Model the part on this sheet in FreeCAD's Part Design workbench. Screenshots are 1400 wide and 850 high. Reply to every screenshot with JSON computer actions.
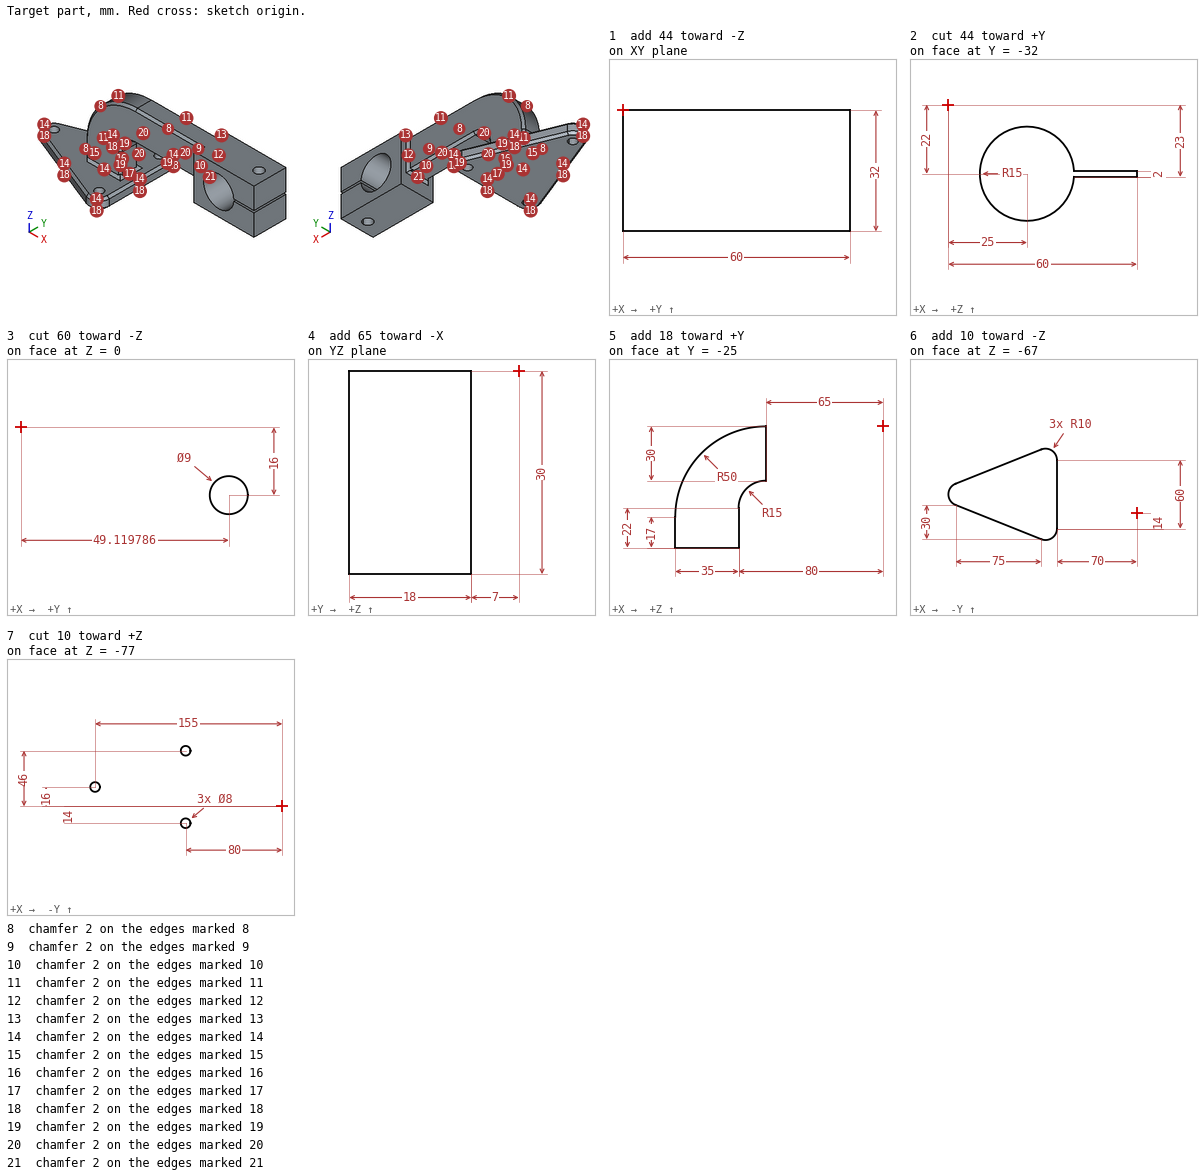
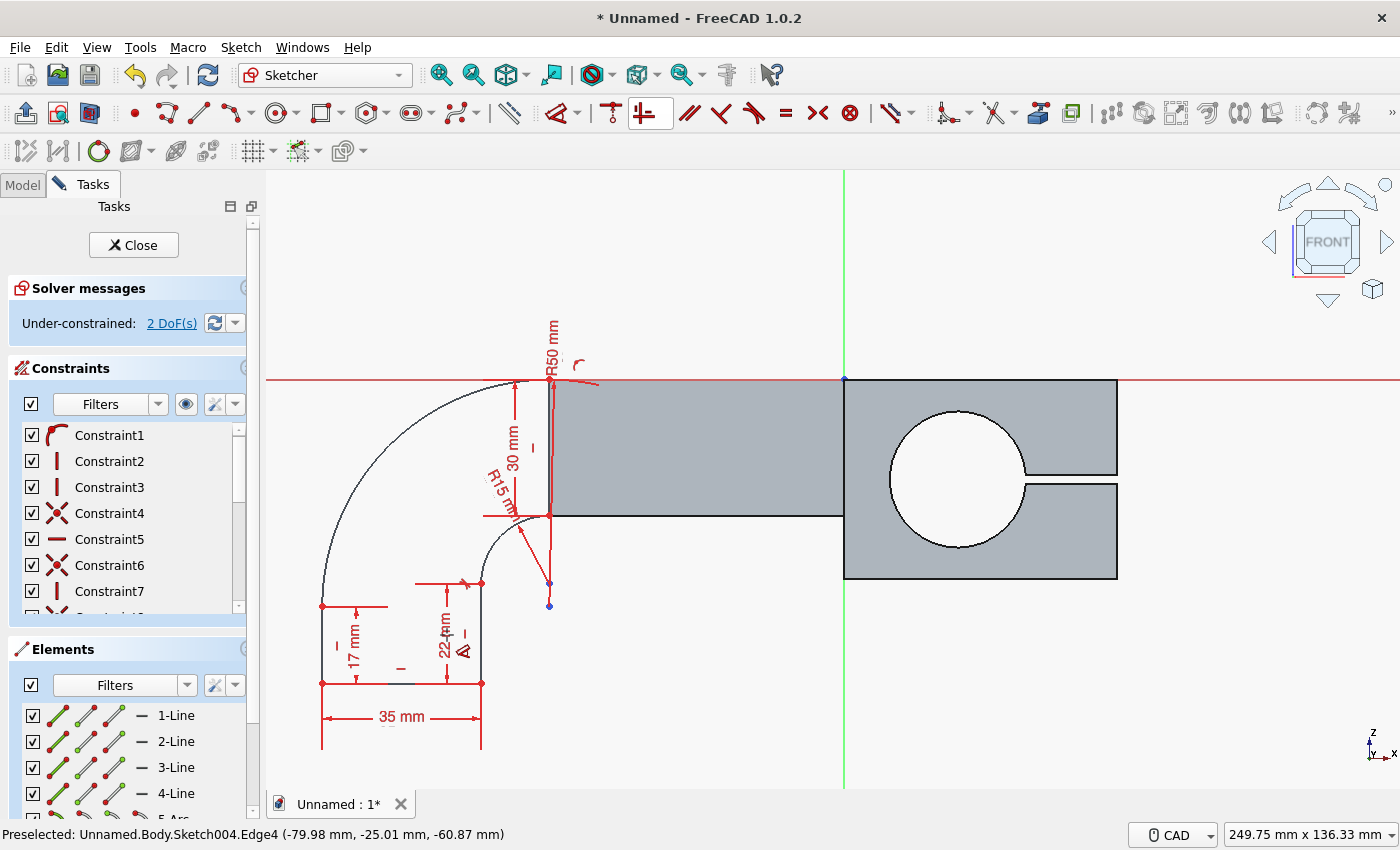
{"action": "left_click", "coordinate": [549, 516]}
{"action": "left_click", "coordinate": [697, 346]}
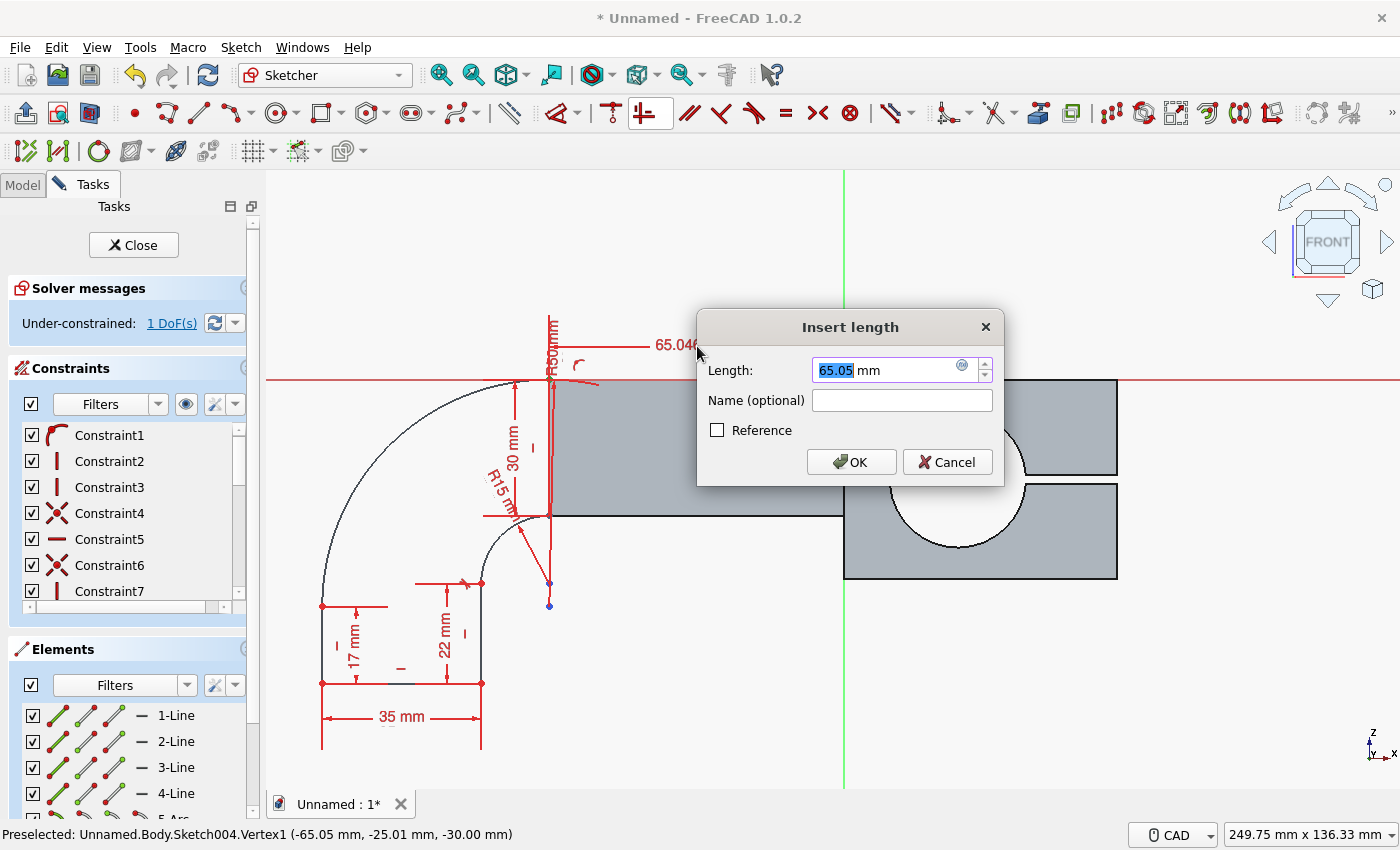
{"action": "type", "text": "65"}
{"action": "key", "text": "Return"}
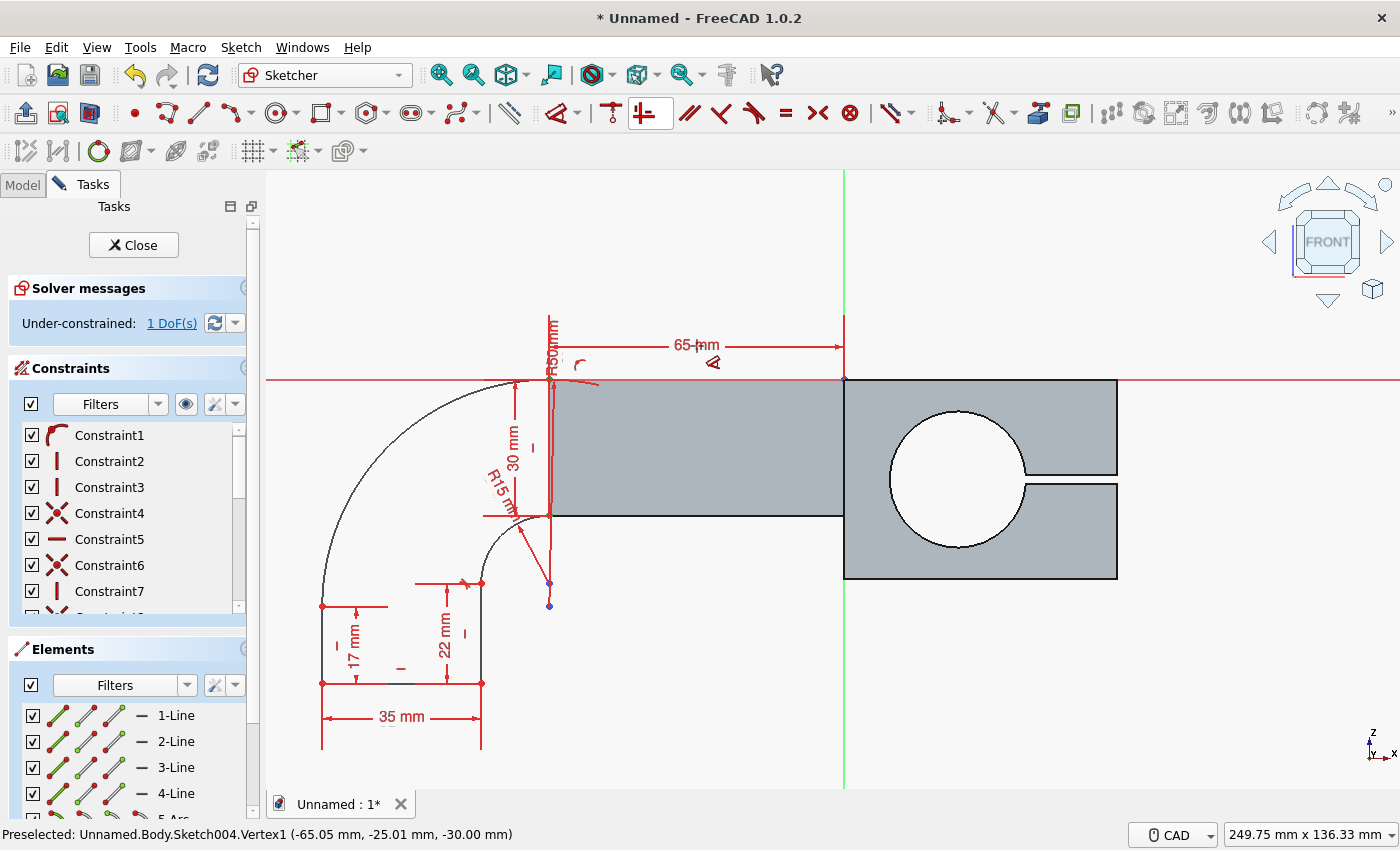
{"action": "left_click", "coordinate": [481, 684]}
{"action": "left_click", "coordinate": [790, 346]}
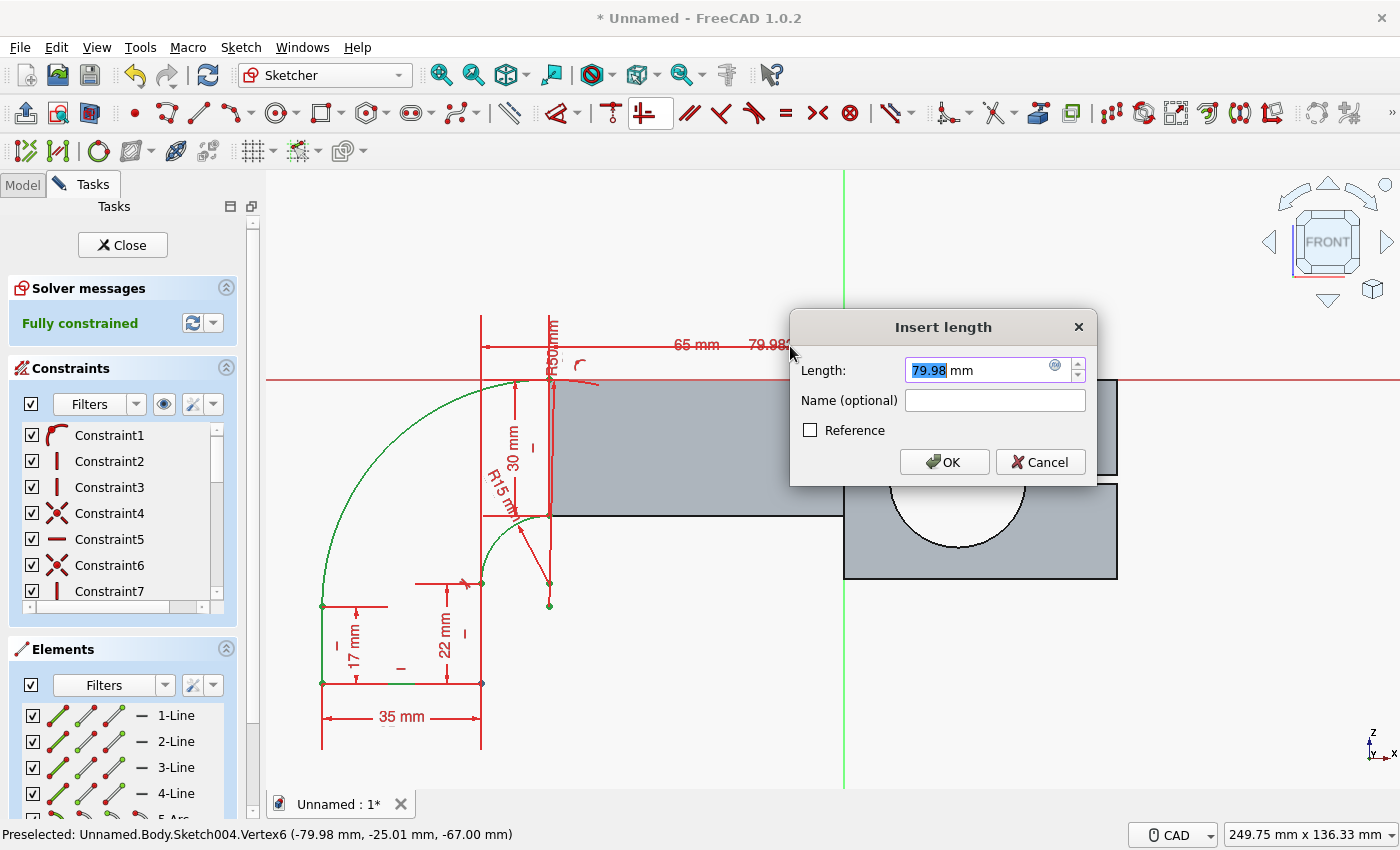
{"action": "type", "text": "80"}
{"action": "key", "text": "Return"}
{"action": "key", "text": "Escape"}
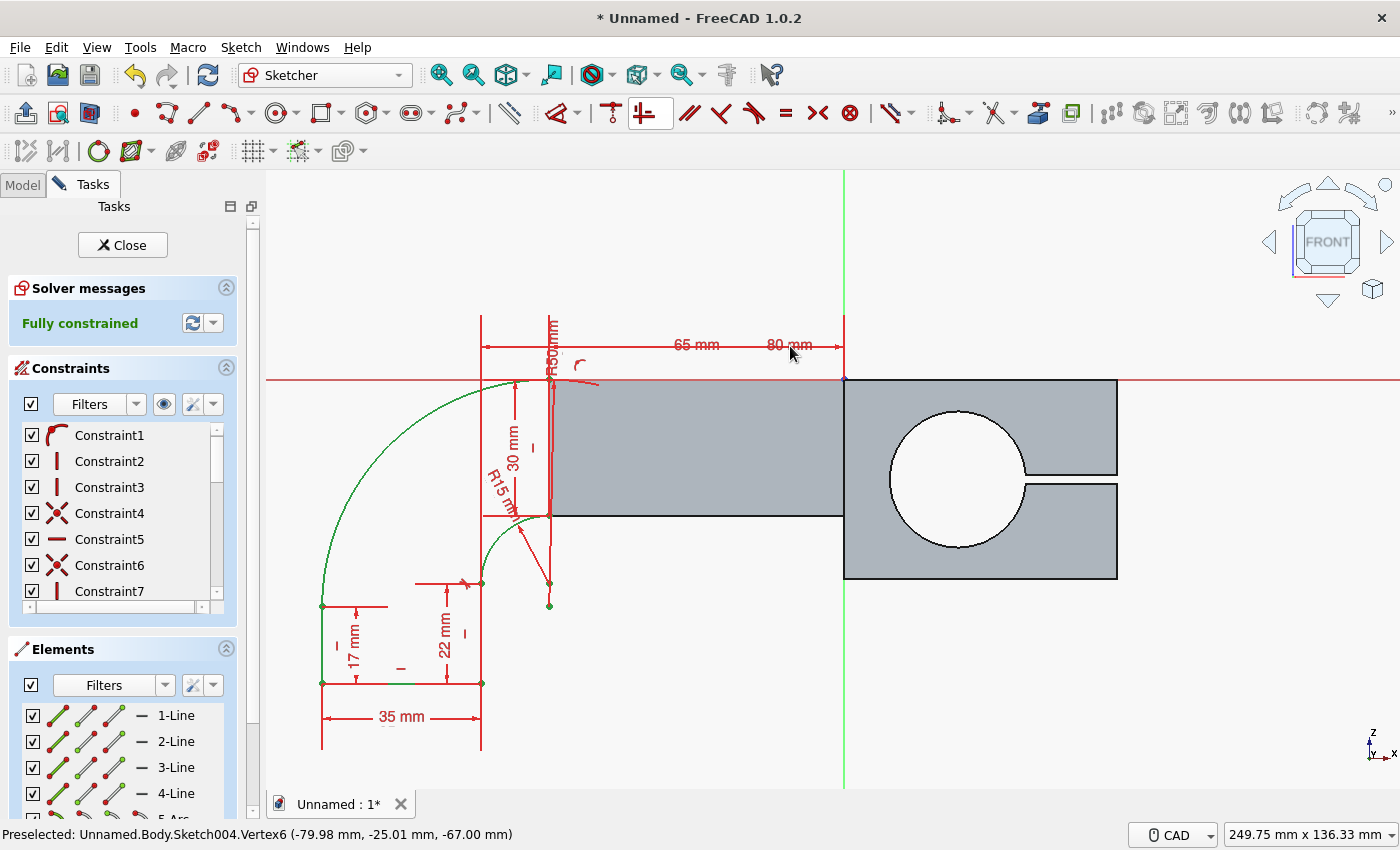
{"action": "left_click", "coordinate": [123, 245]}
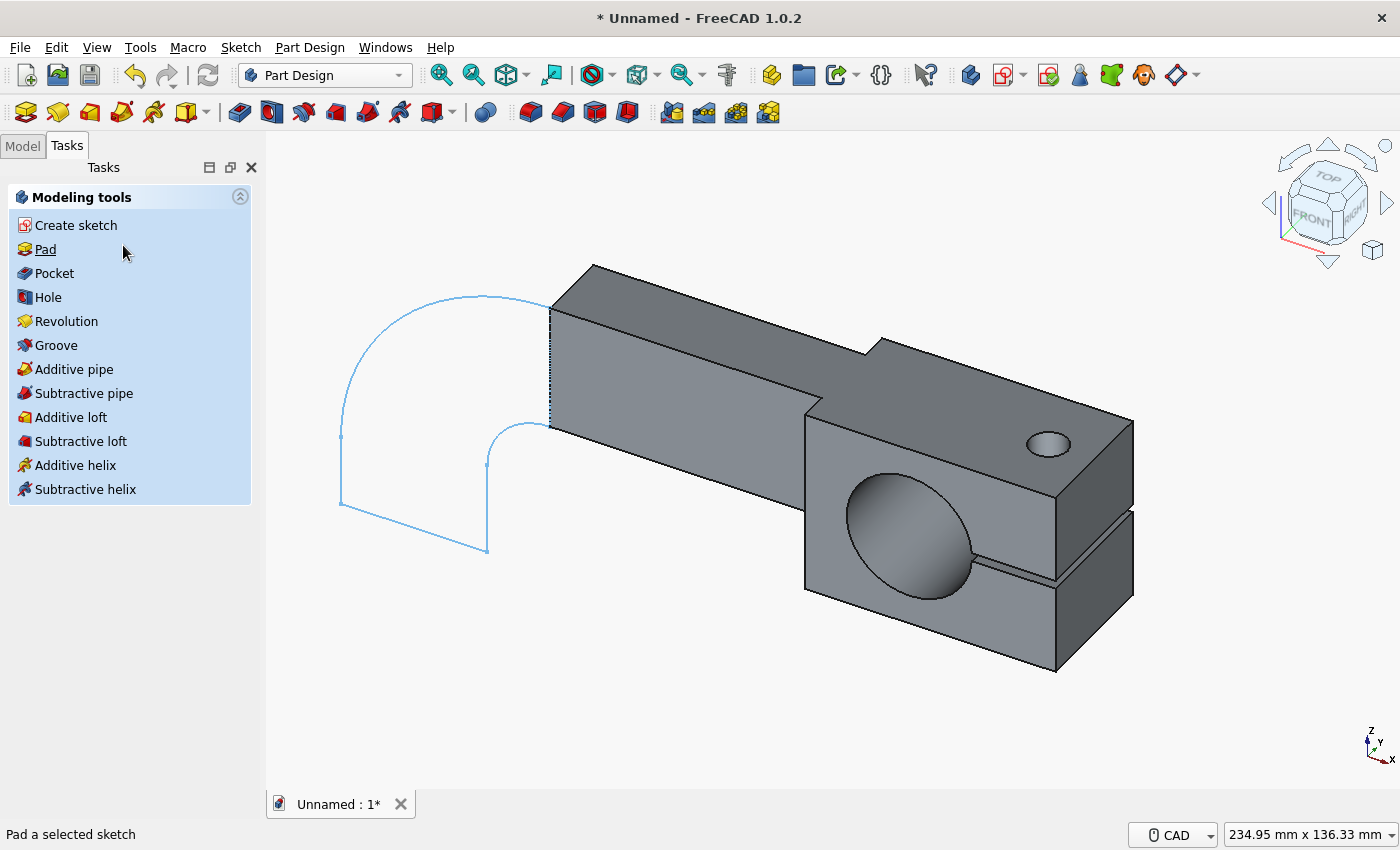
{"action": "left_click", "coordinate": [26, 112]}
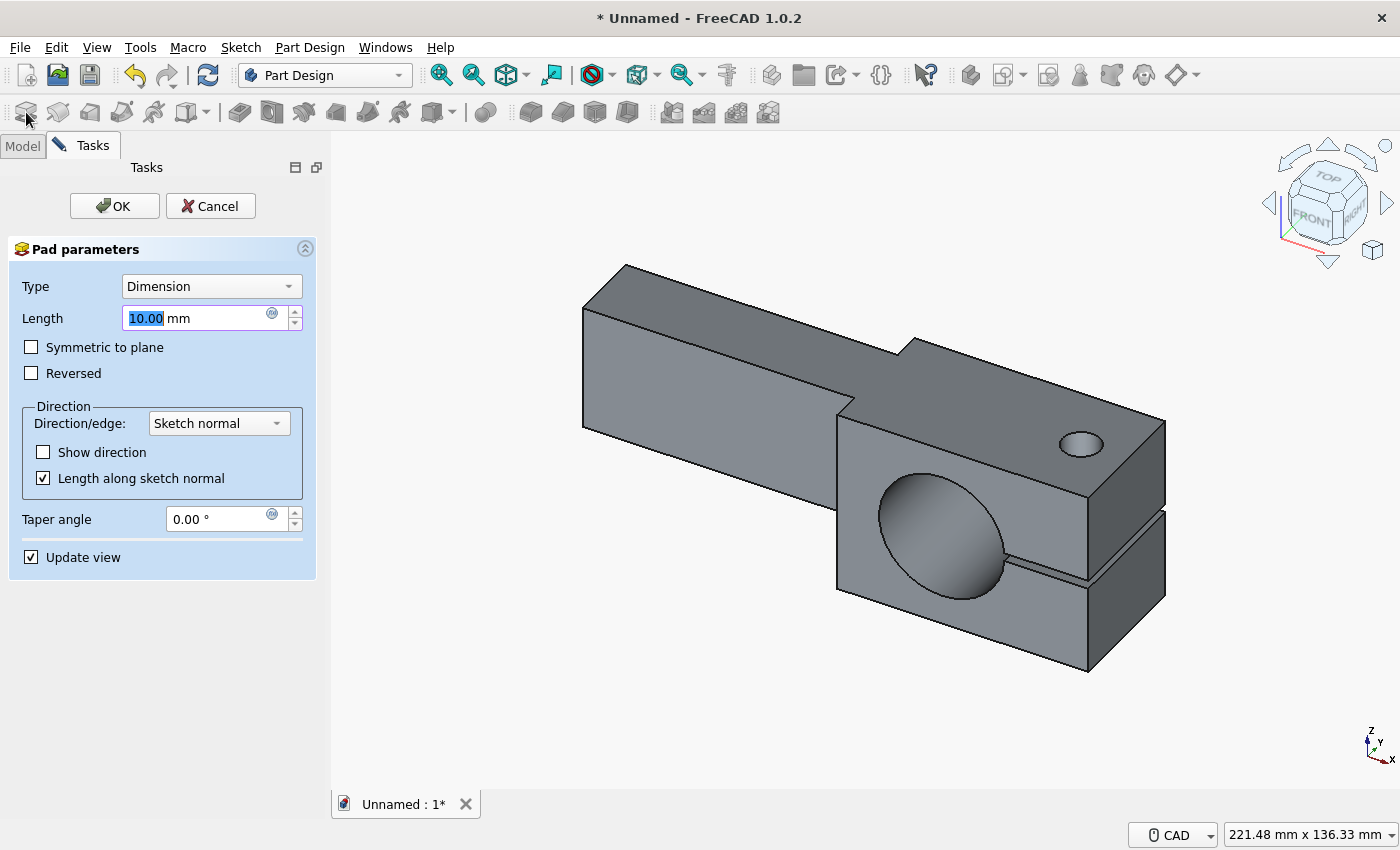
{"action": "type", "text": "18"}
{"action": "key", "text": "Tab"}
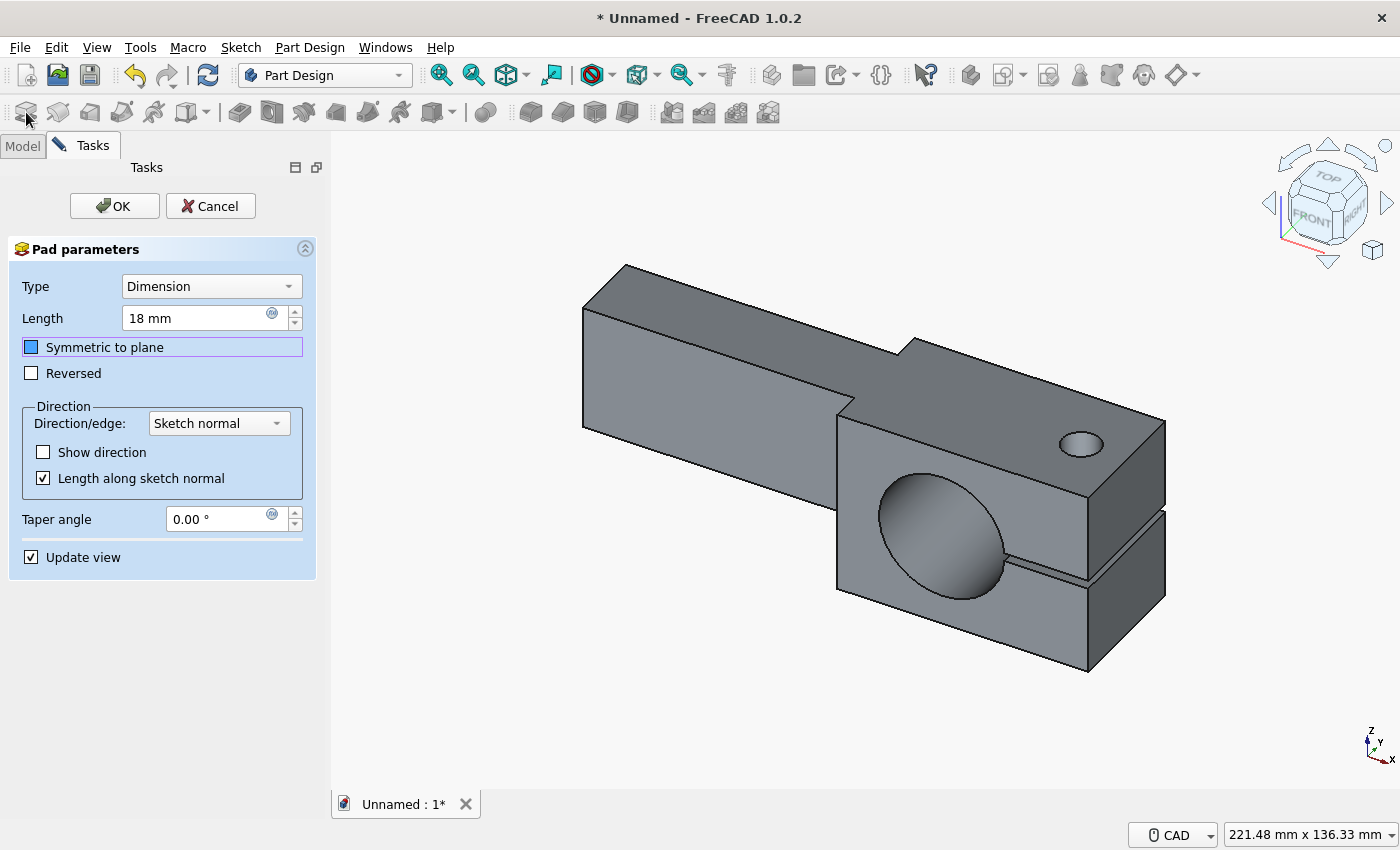
{"action": "left_click", "coordinate": [30, 373]}